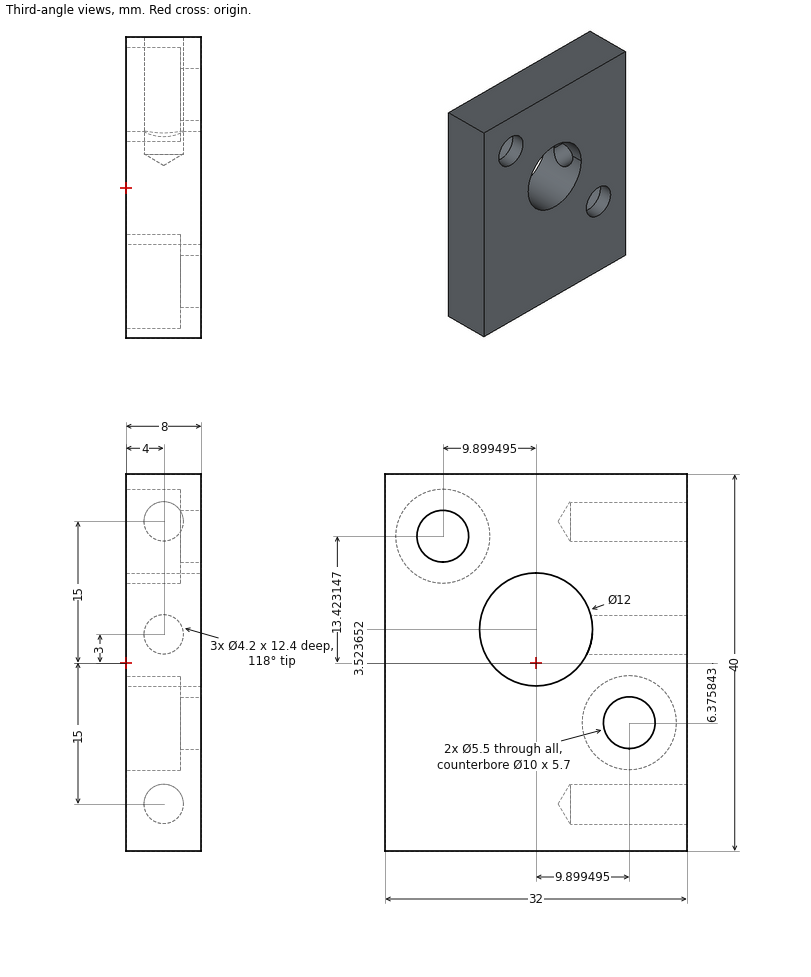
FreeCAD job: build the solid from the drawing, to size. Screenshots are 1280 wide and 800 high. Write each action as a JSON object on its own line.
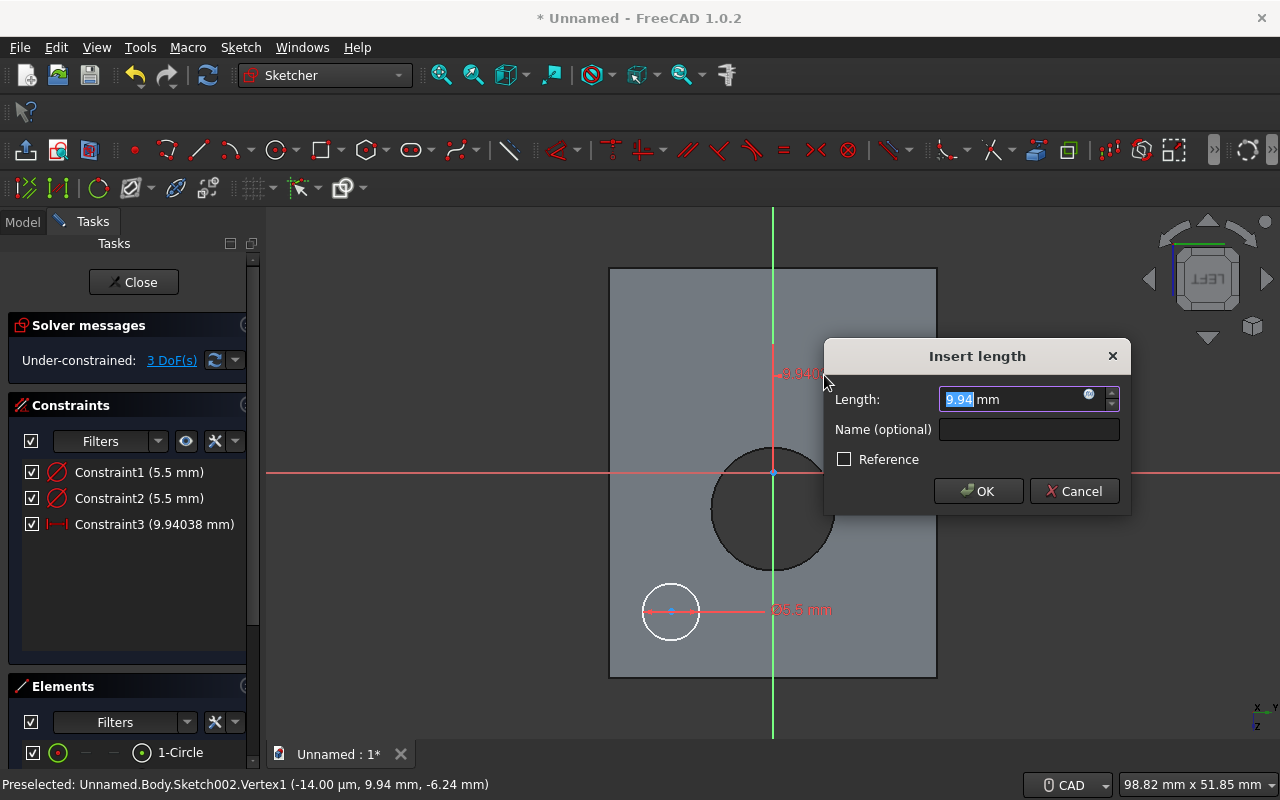
{"action": "type", "text": "9.899495"}
{"action": "key", "text": "Return"}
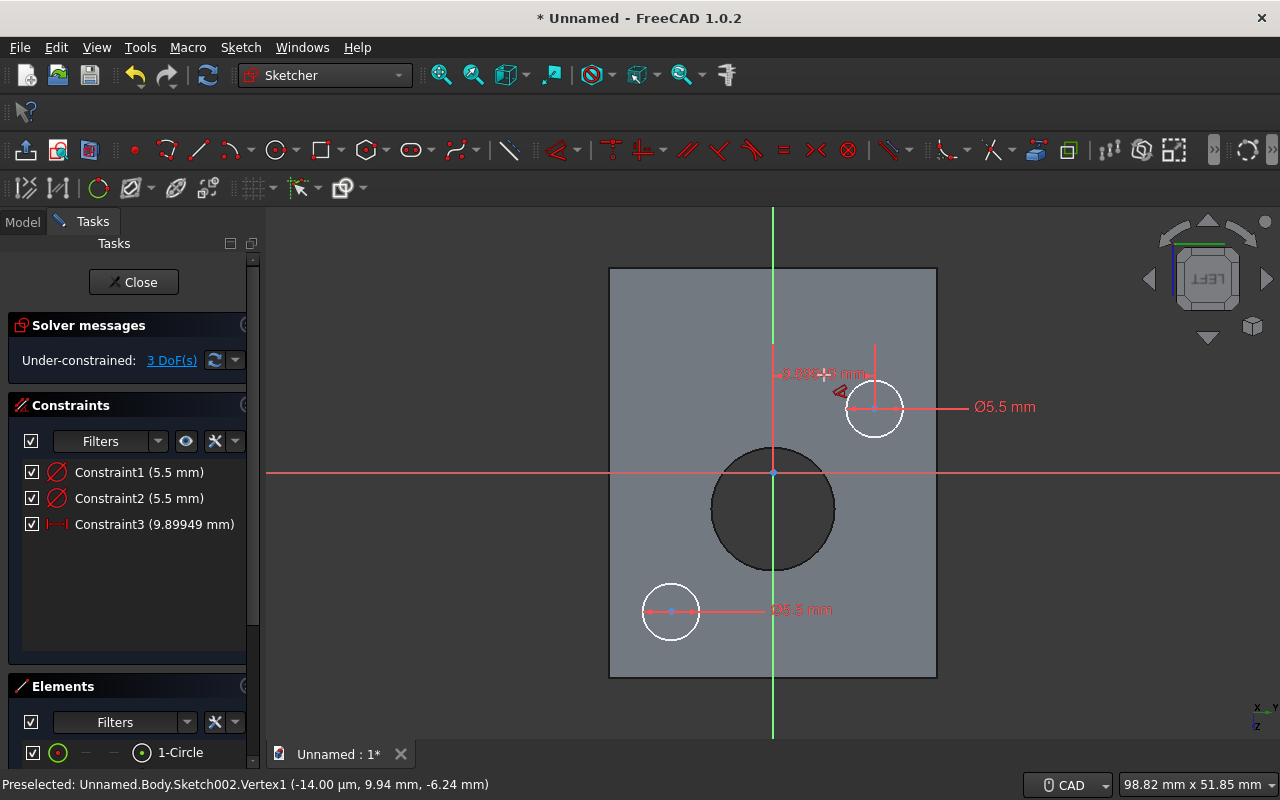
{"action": "left_click", "coordinate": [875, 409]}
{"action": "left_click", "coordinate": [909, 441]}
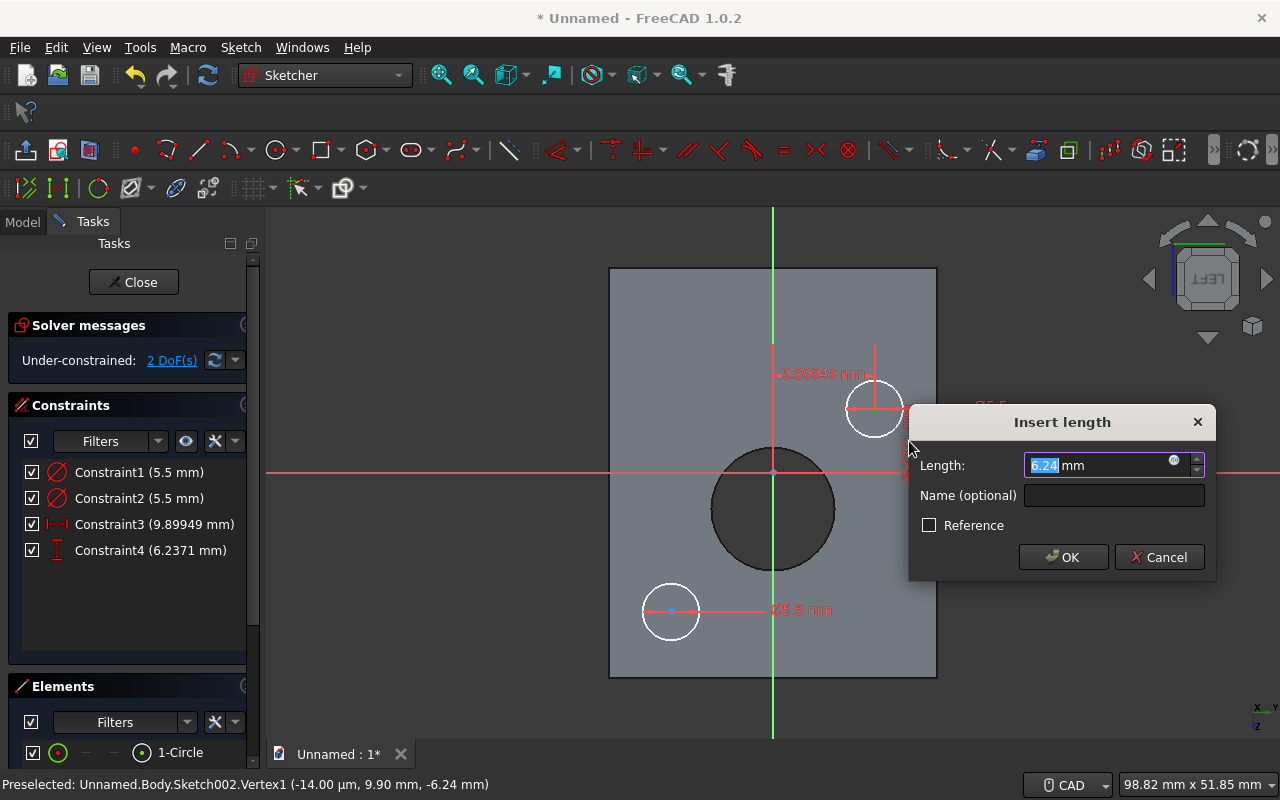
{"action": "type", "text": "6.375843"}
{"action": "key", "text": "Return"}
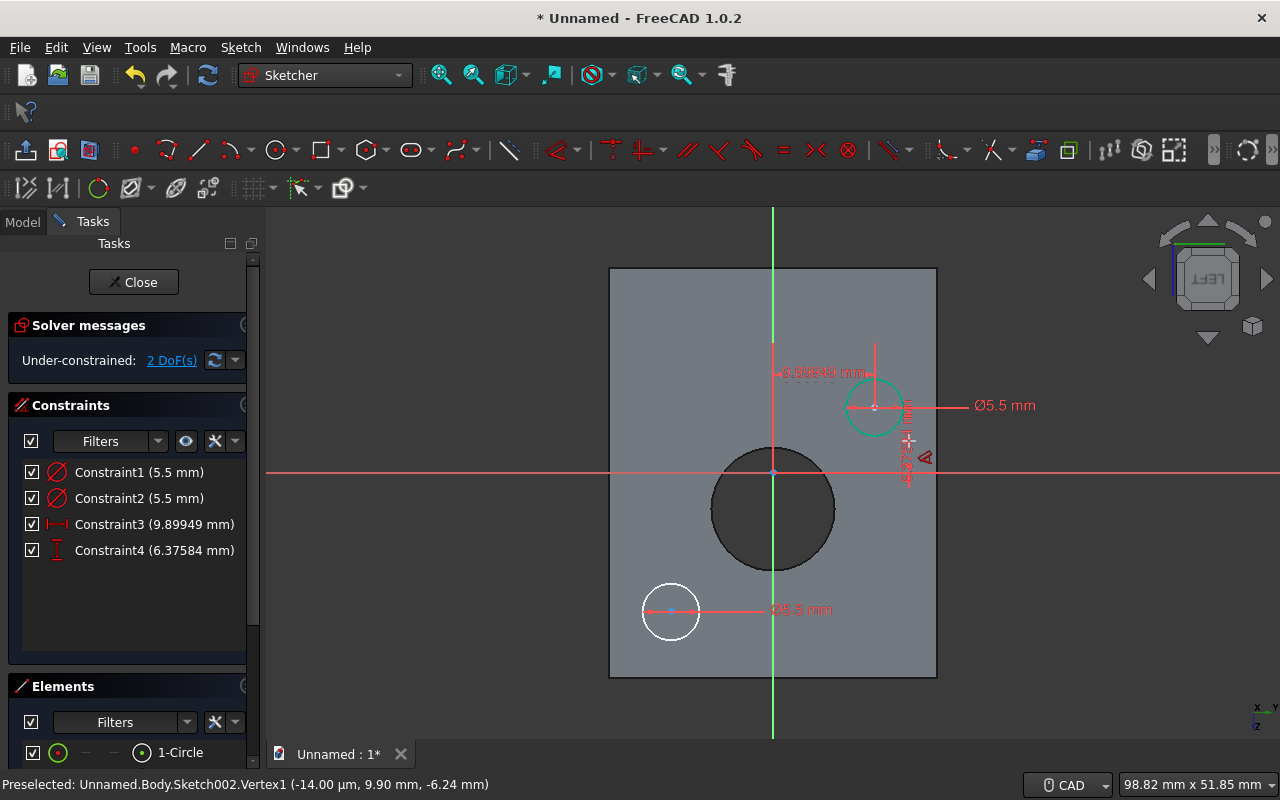
{"action": "left_click", "coordinate": [671, 612]}
{"action": "left_click", "coordinate": [722, 646]}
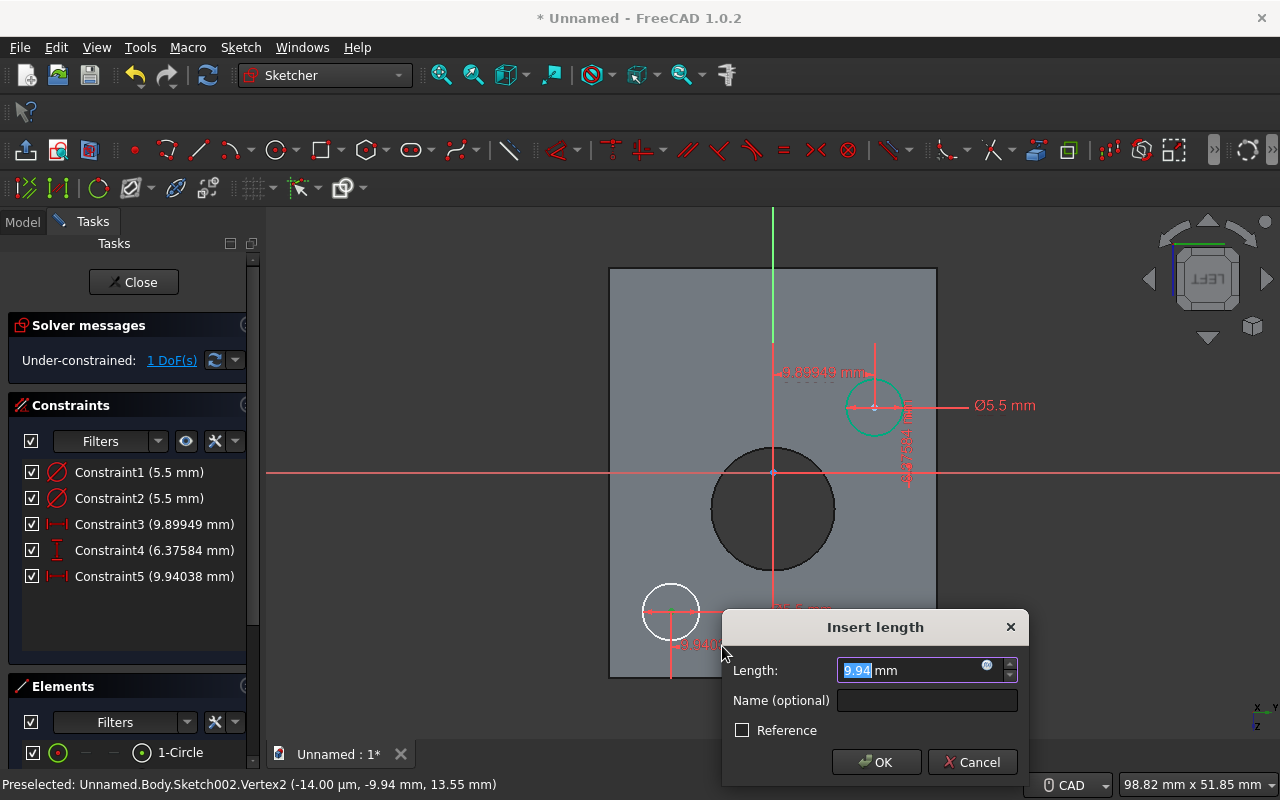
{"action": "type", "text": "9.899495"}
{"action": "key", "text": "Return"}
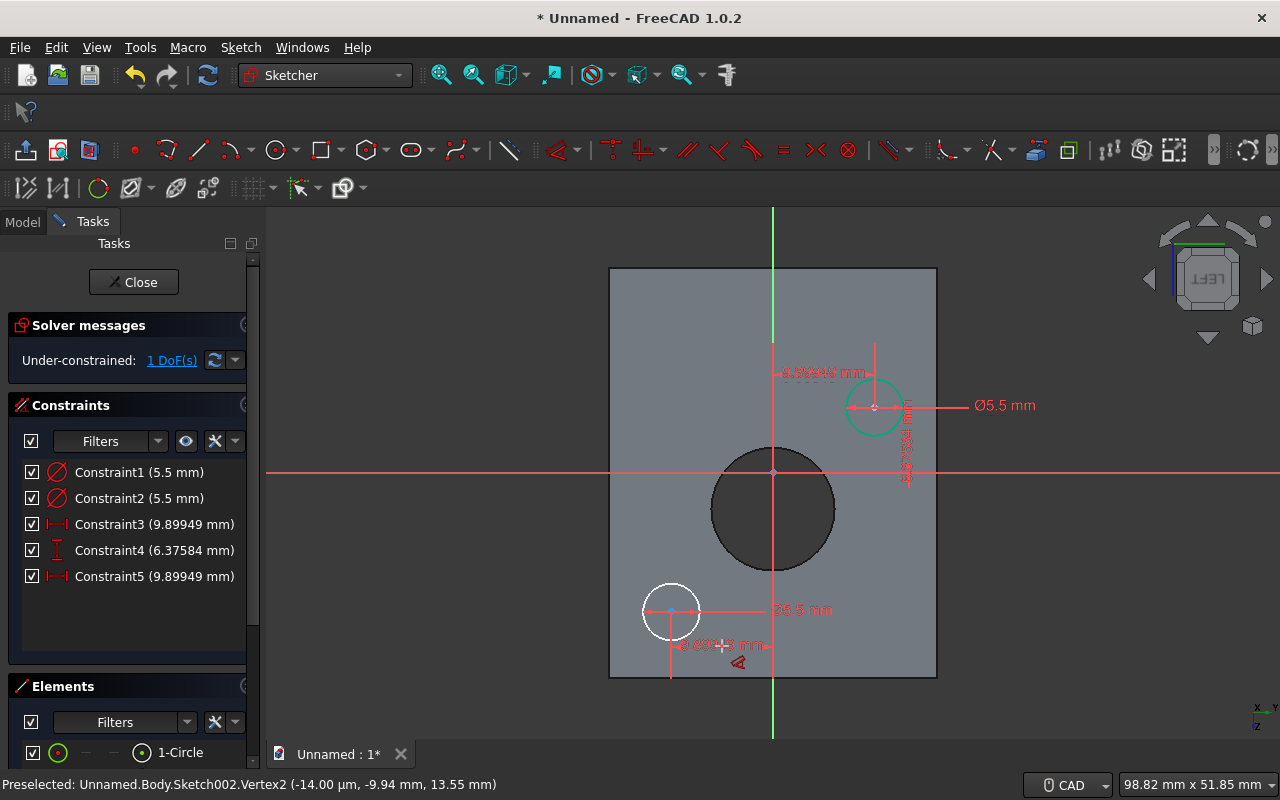
{"action": "left_click", "coordinate": [671, 612]}
{"action": "left_click", "coordinate": [637, 542]}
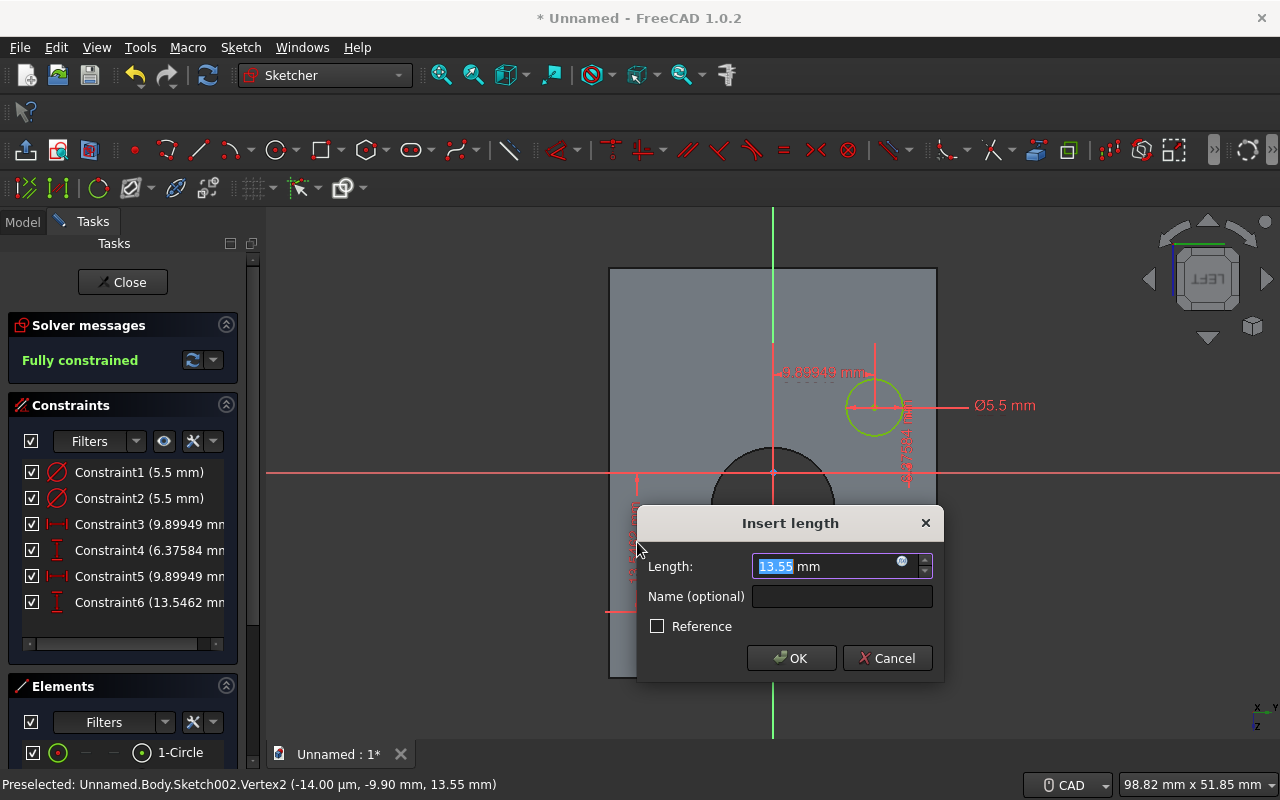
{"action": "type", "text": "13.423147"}
{"action": "key", "text": "Return"}
{"action": "key", "text": "Escape"}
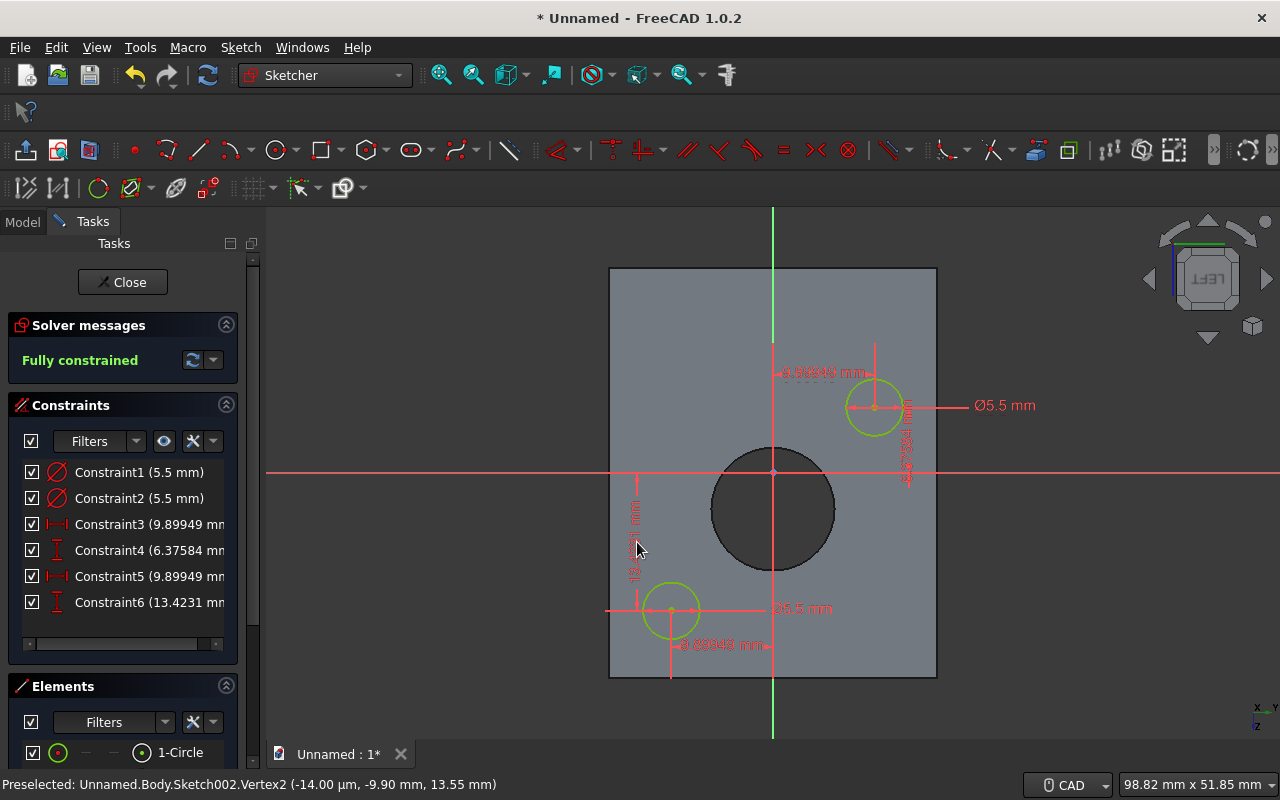
{"action": "left_click", "coordinate": [123, 282]}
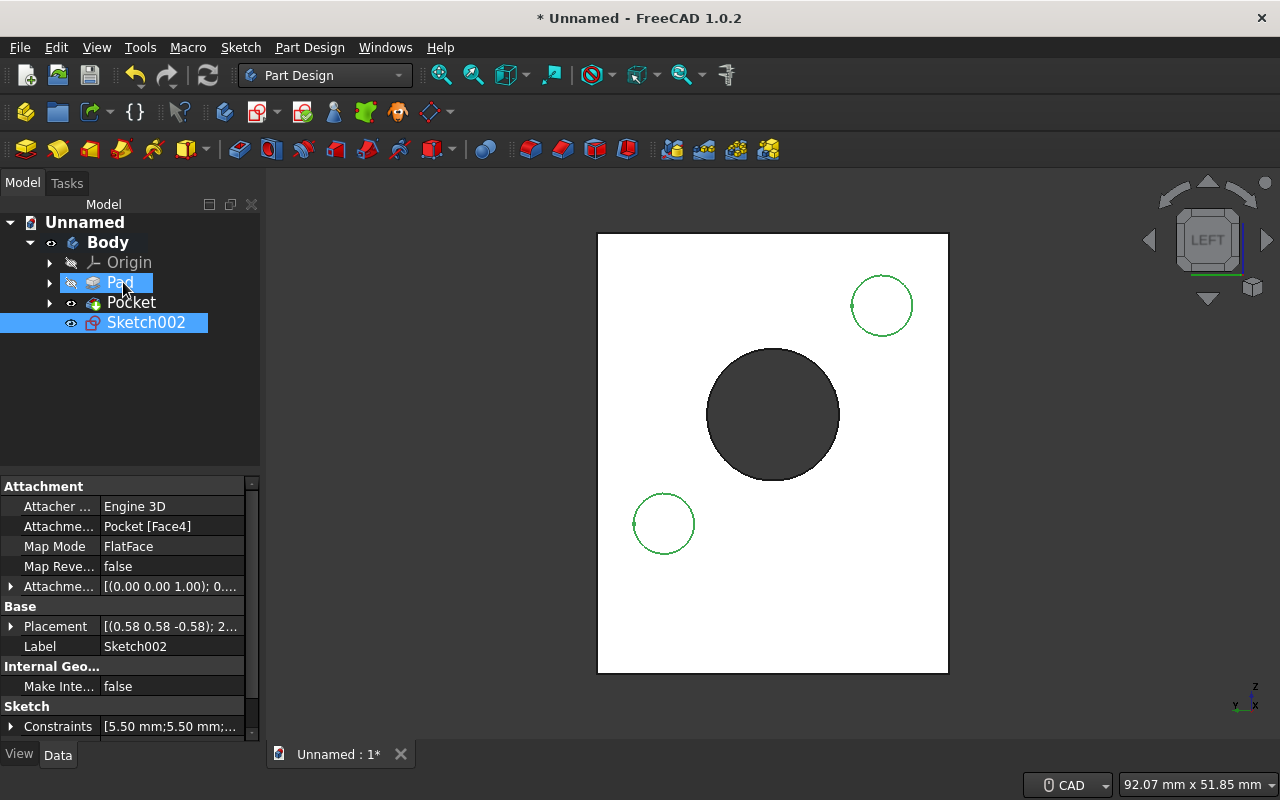
{"action": "left_click", "coordinate": [272, 150]}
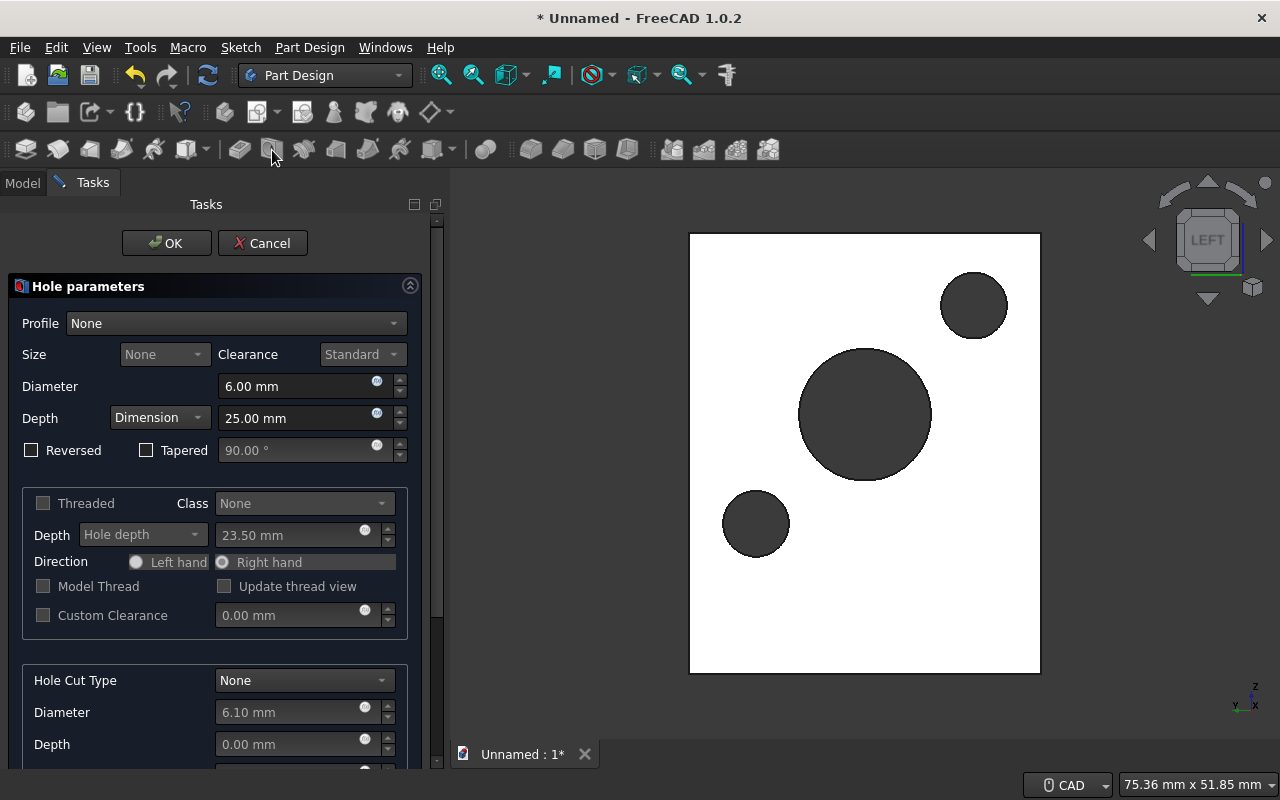
{"action": "triple_click", "coordinate": [305, 386]}